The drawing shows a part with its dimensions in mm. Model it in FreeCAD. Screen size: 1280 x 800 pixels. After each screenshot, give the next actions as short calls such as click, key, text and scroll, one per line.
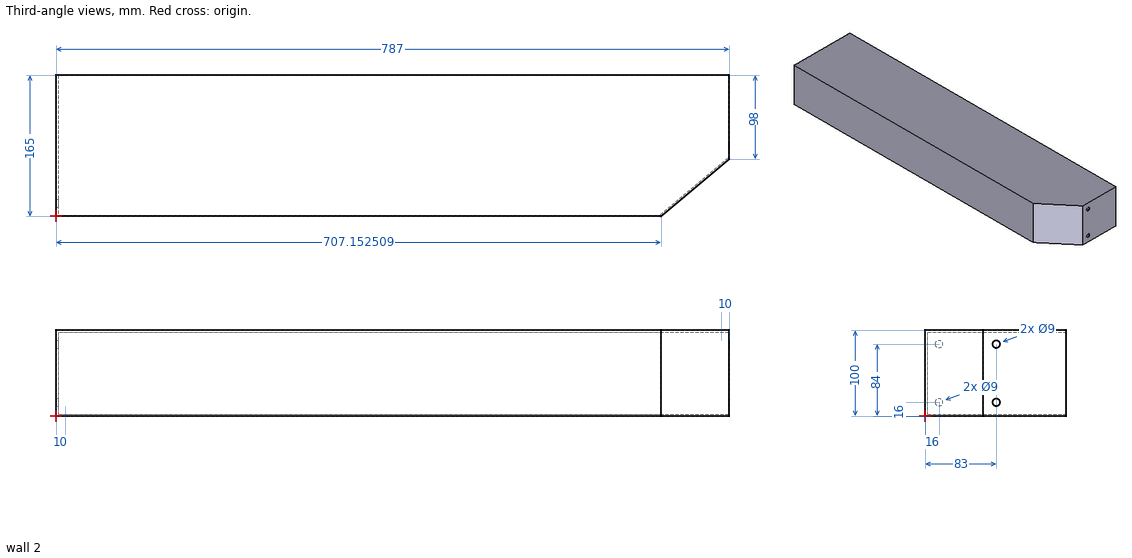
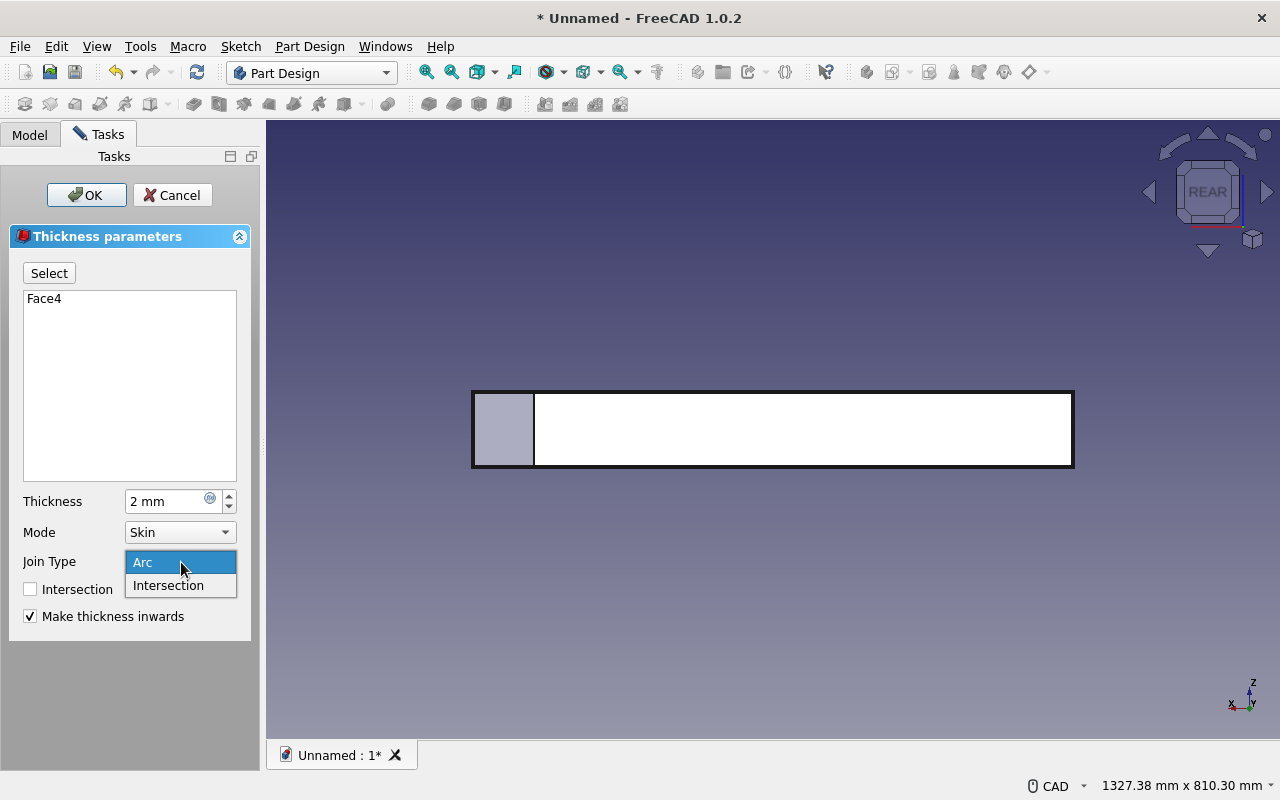
click(179, 586)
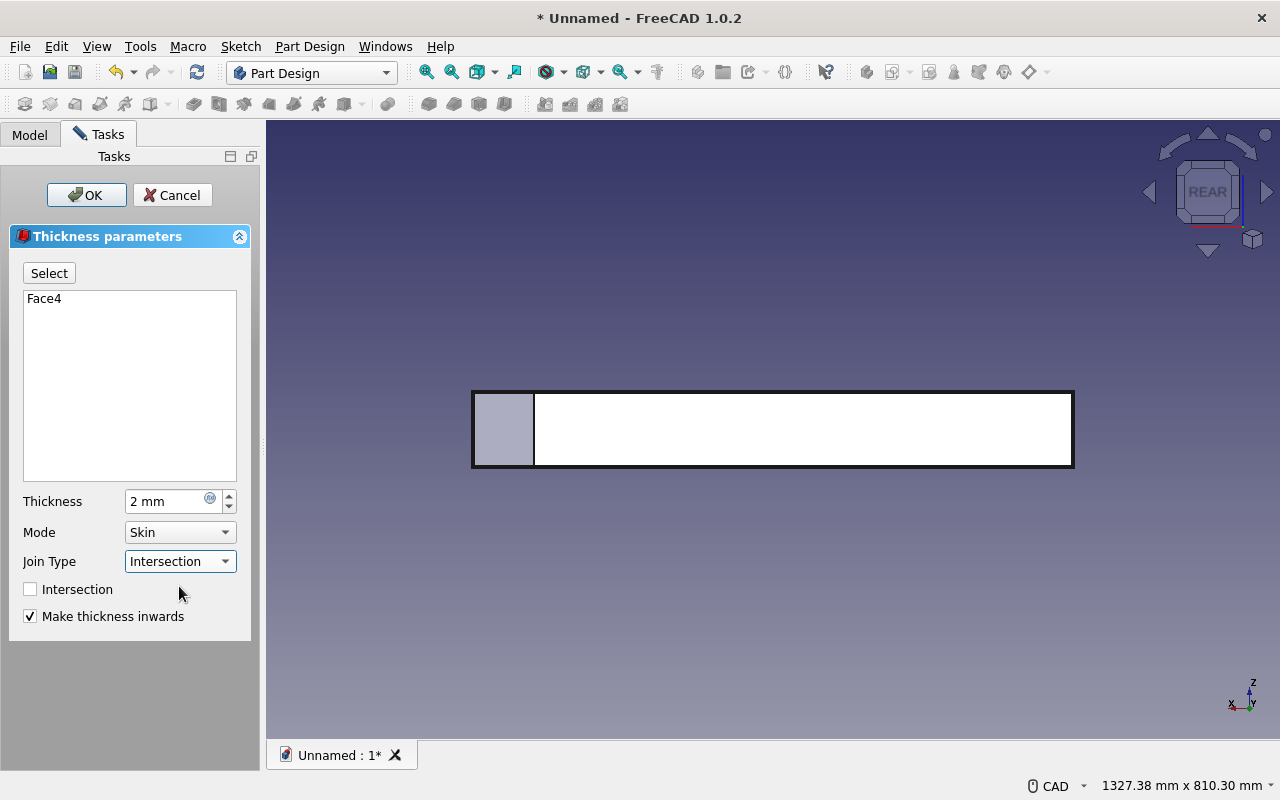
click(87, 195)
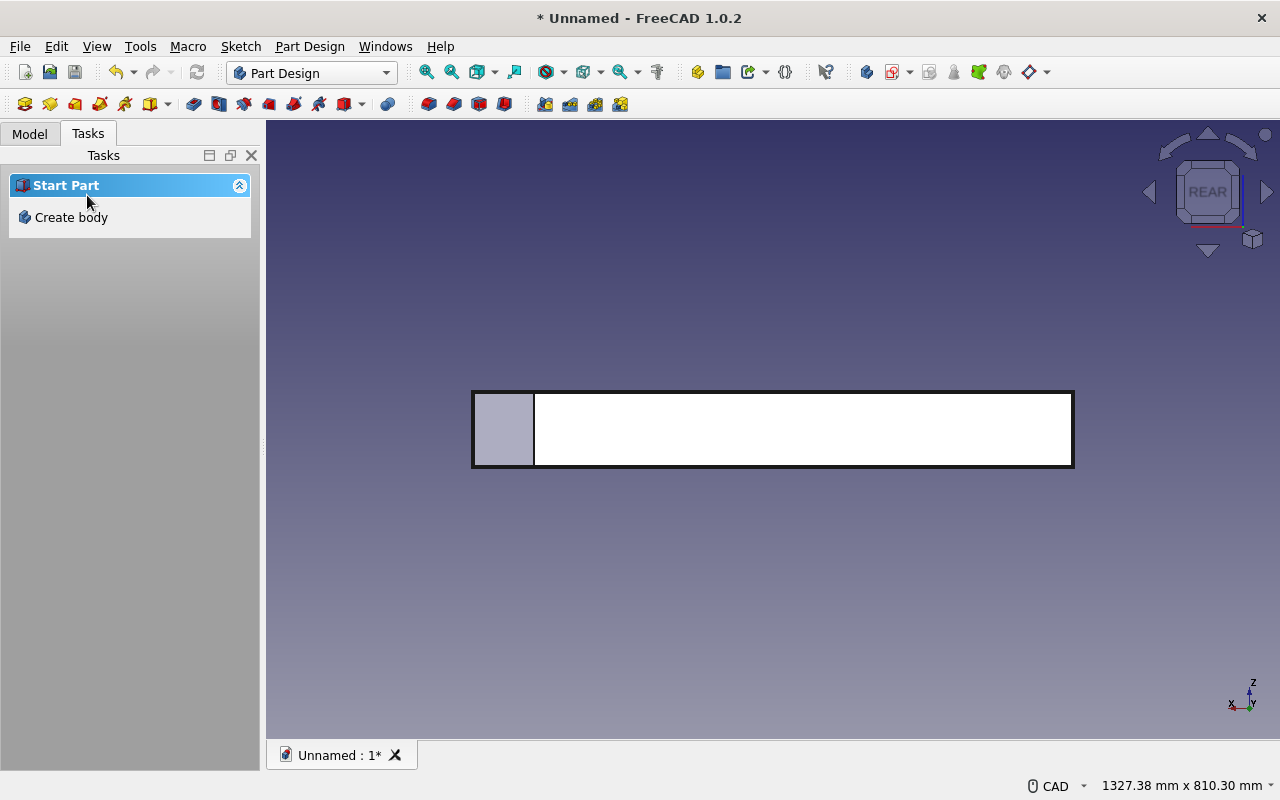
click(892, 72)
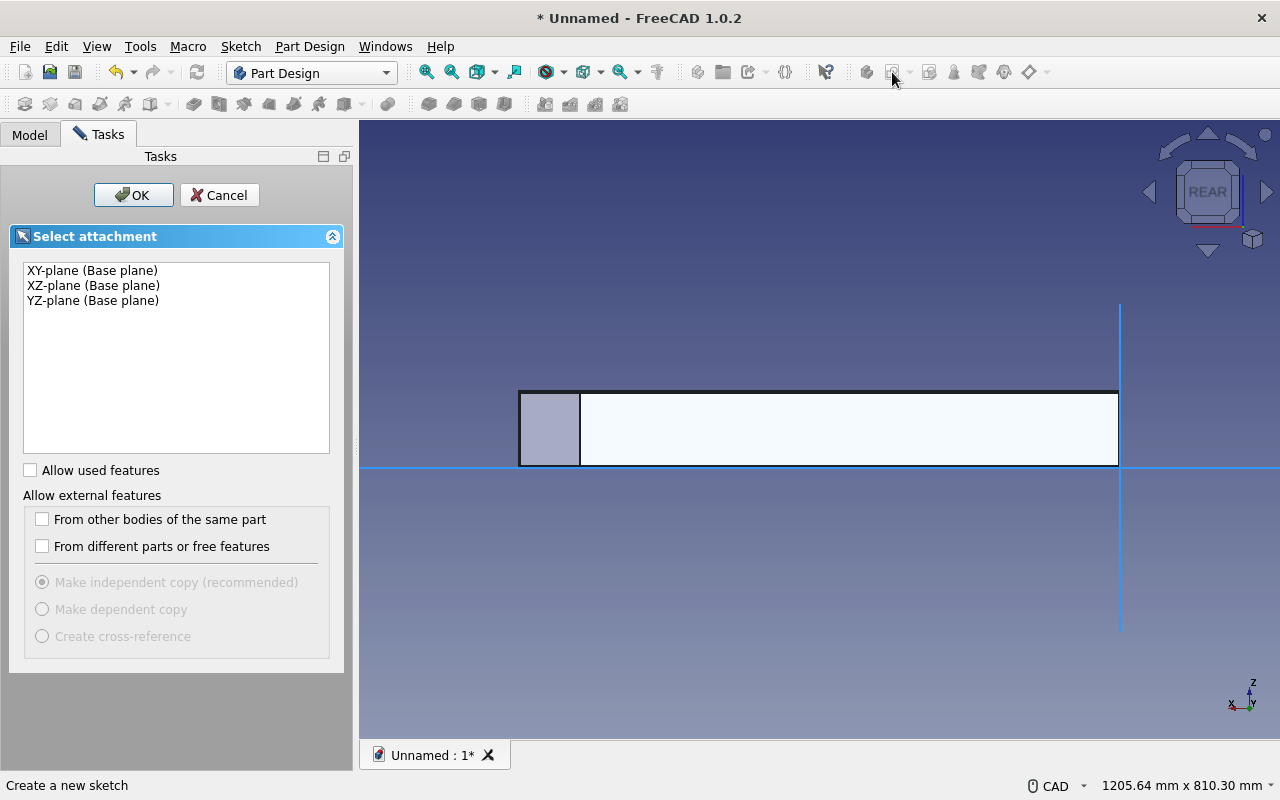
click(84, 300)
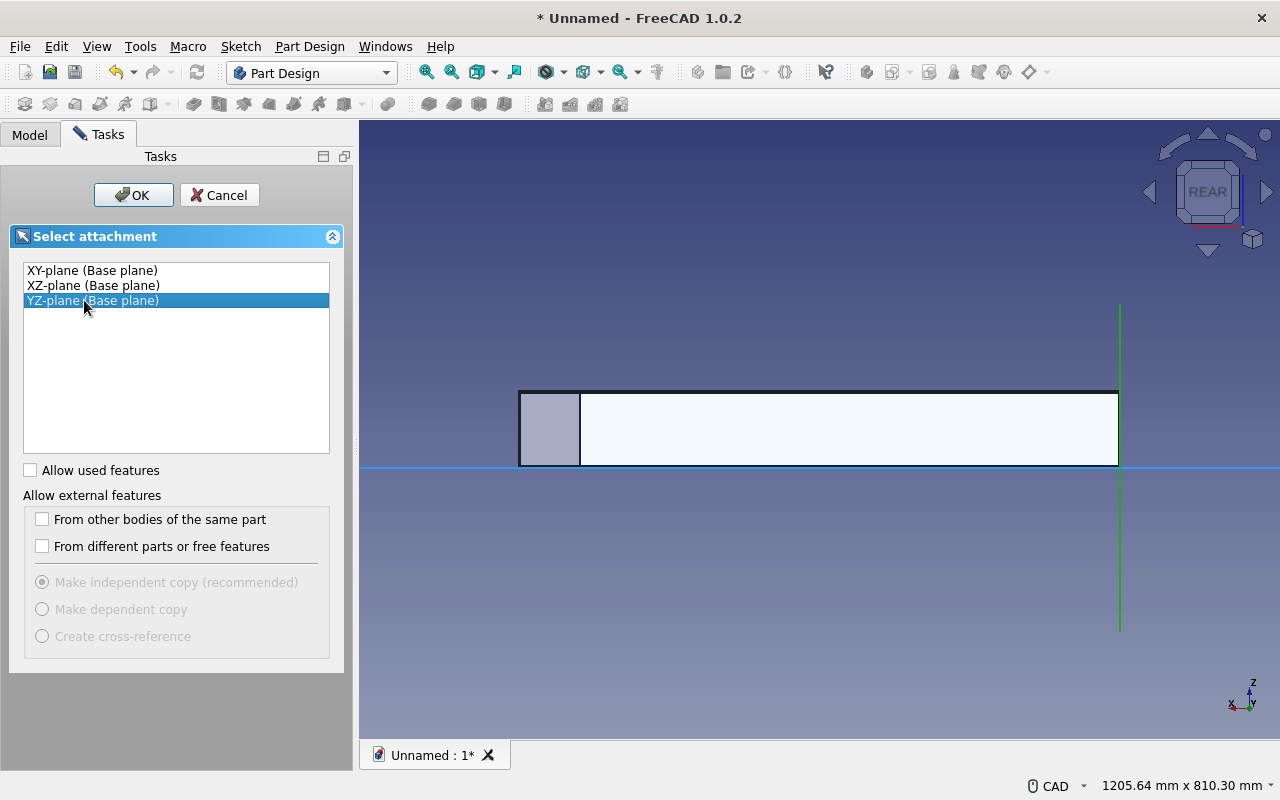
click(134, 195)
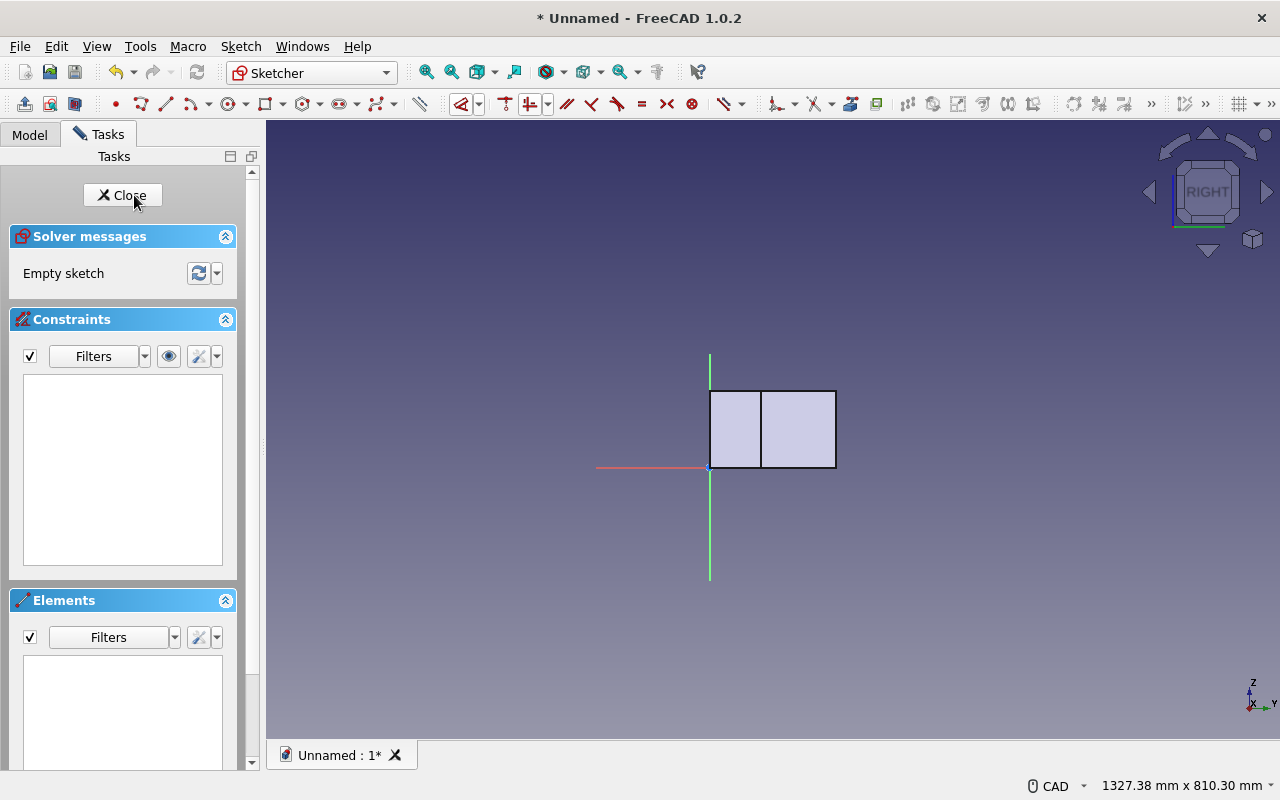
click(75, 104)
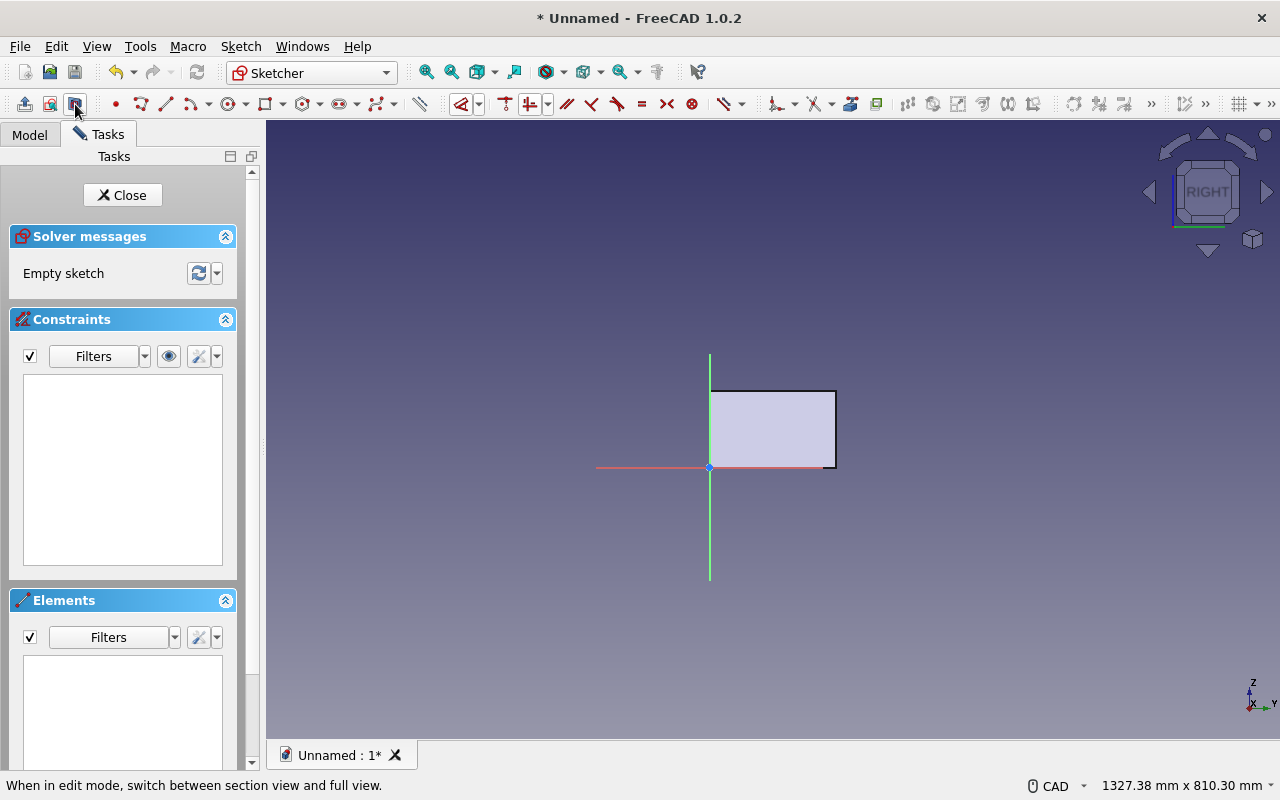
scroll(720, 435, up, 9)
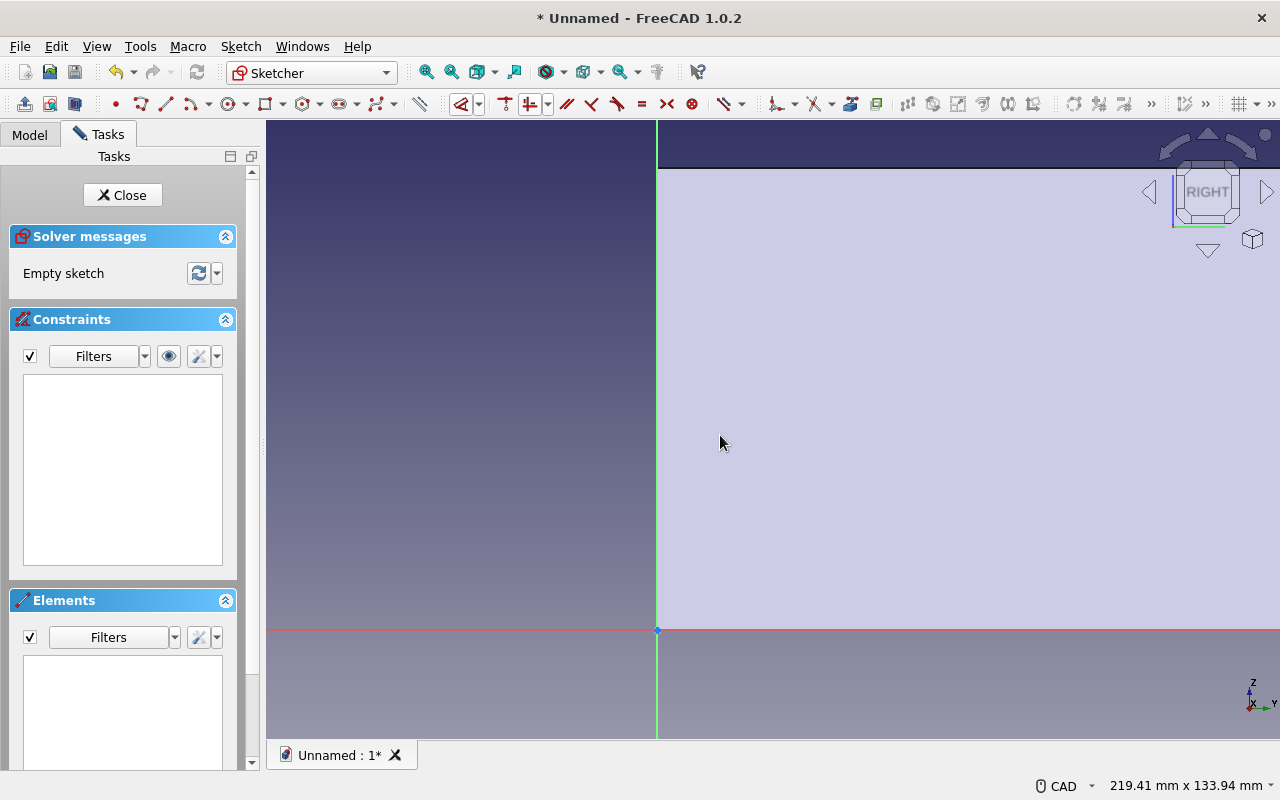
click(228, 104)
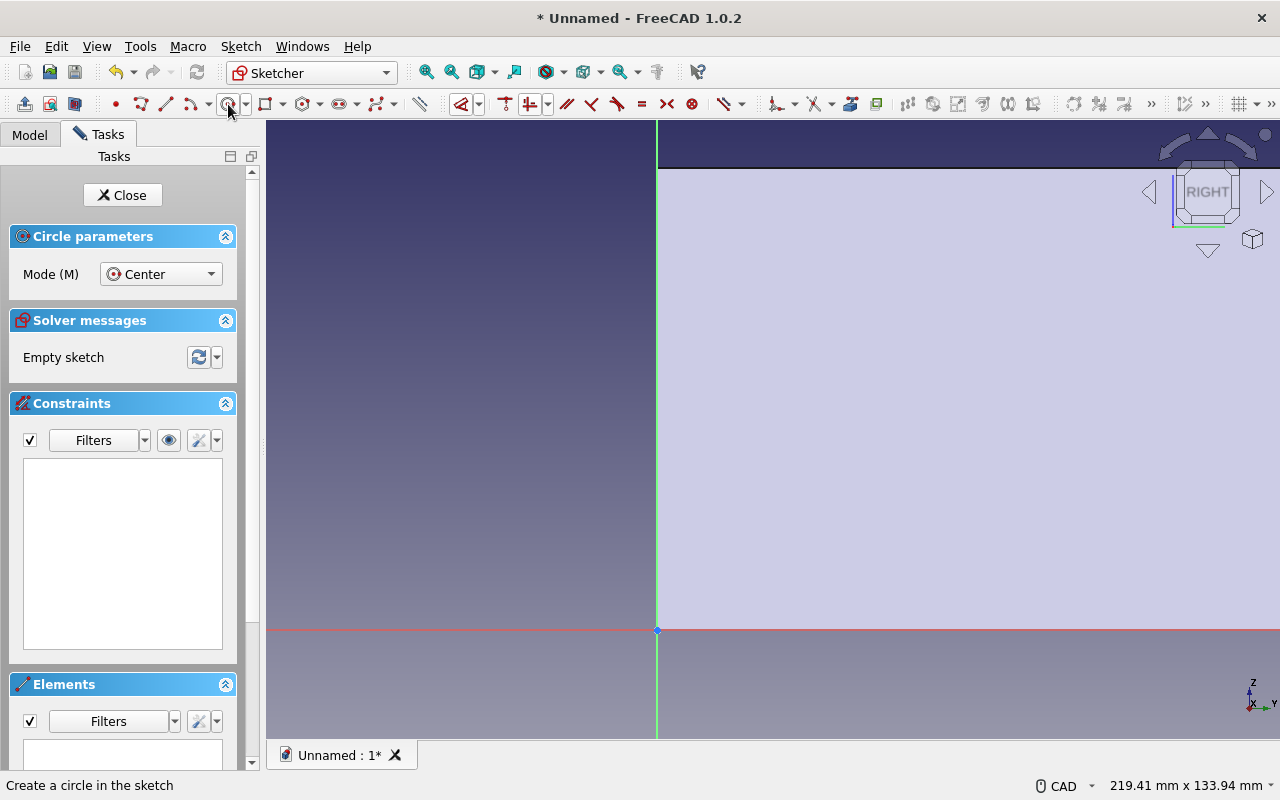
click(731, 556)
move(746, 542)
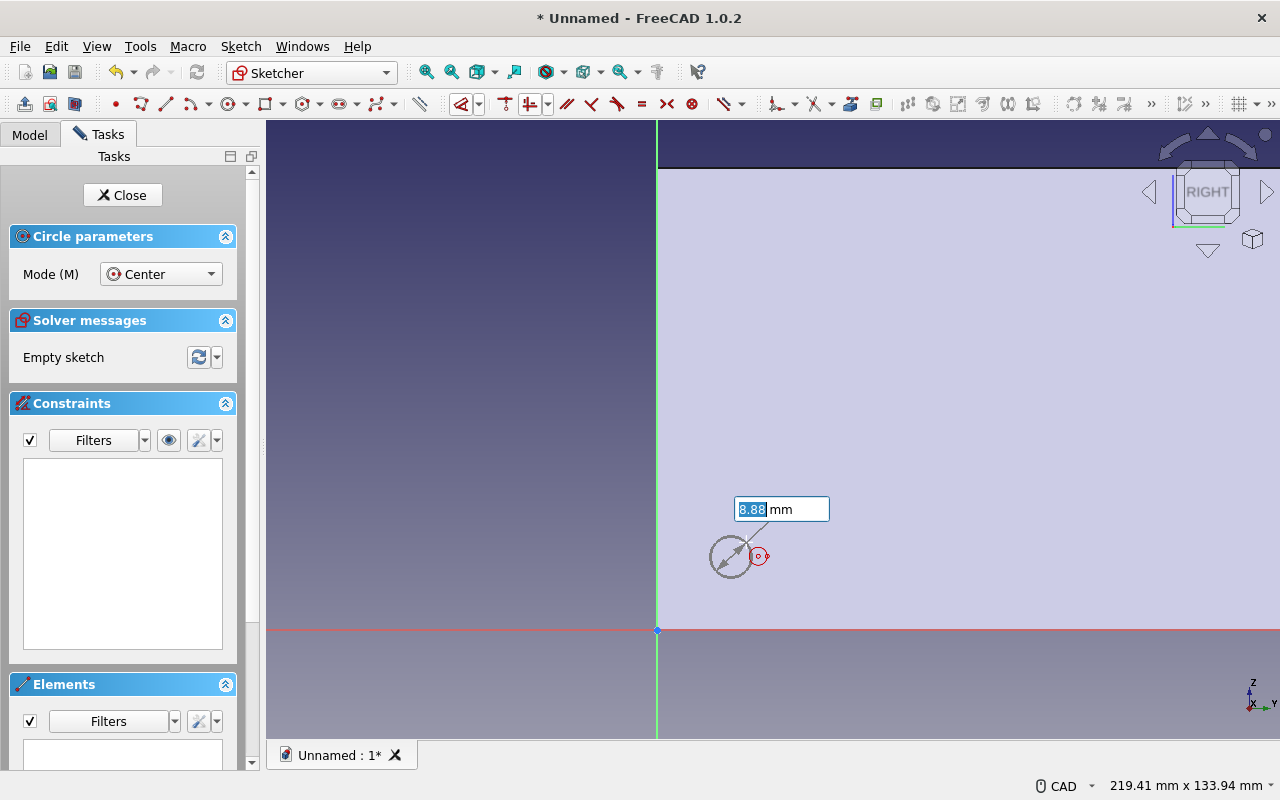
text(9)
key(Return)